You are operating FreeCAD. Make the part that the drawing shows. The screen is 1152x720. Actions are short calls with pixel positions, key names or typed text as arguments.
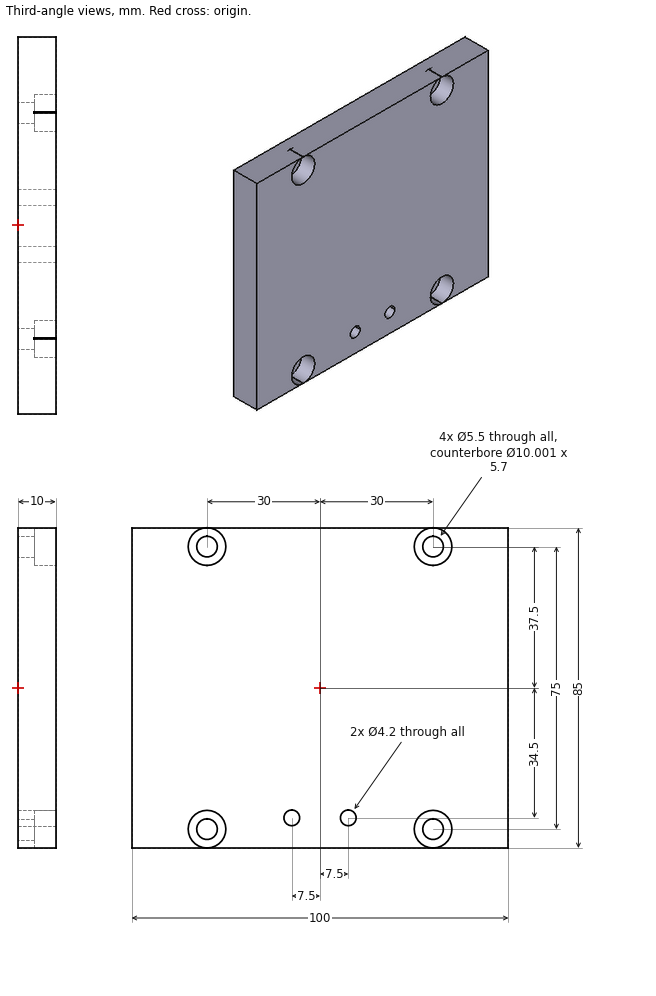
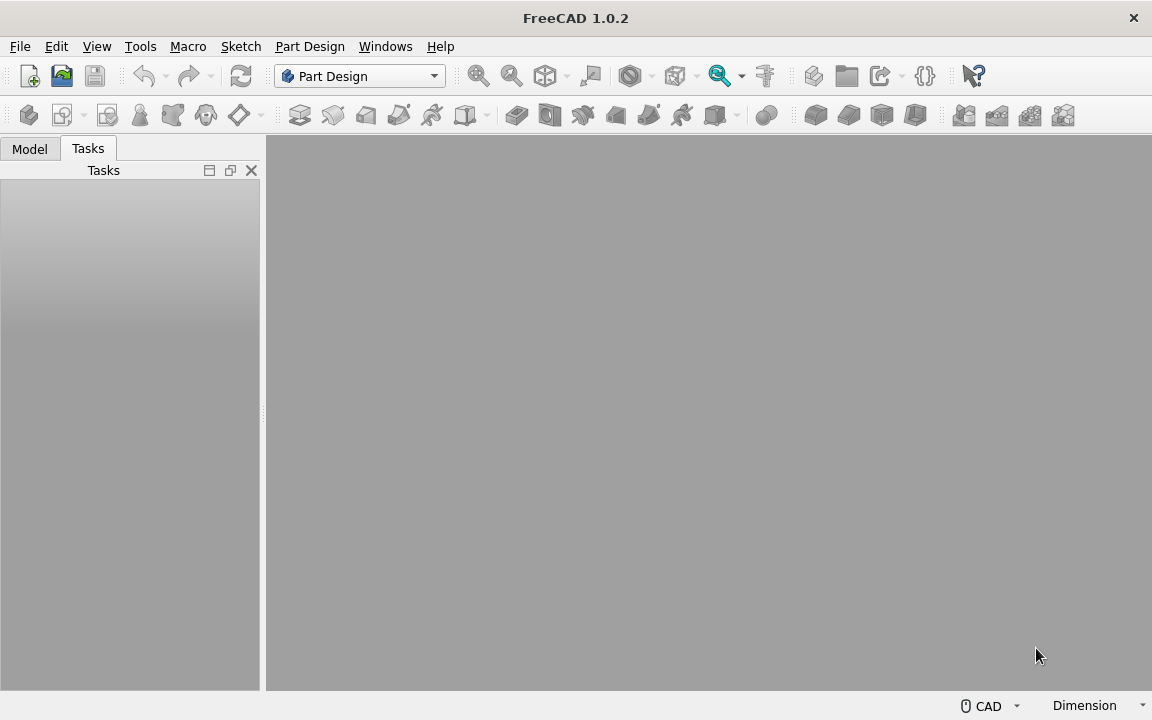
click(29, 76)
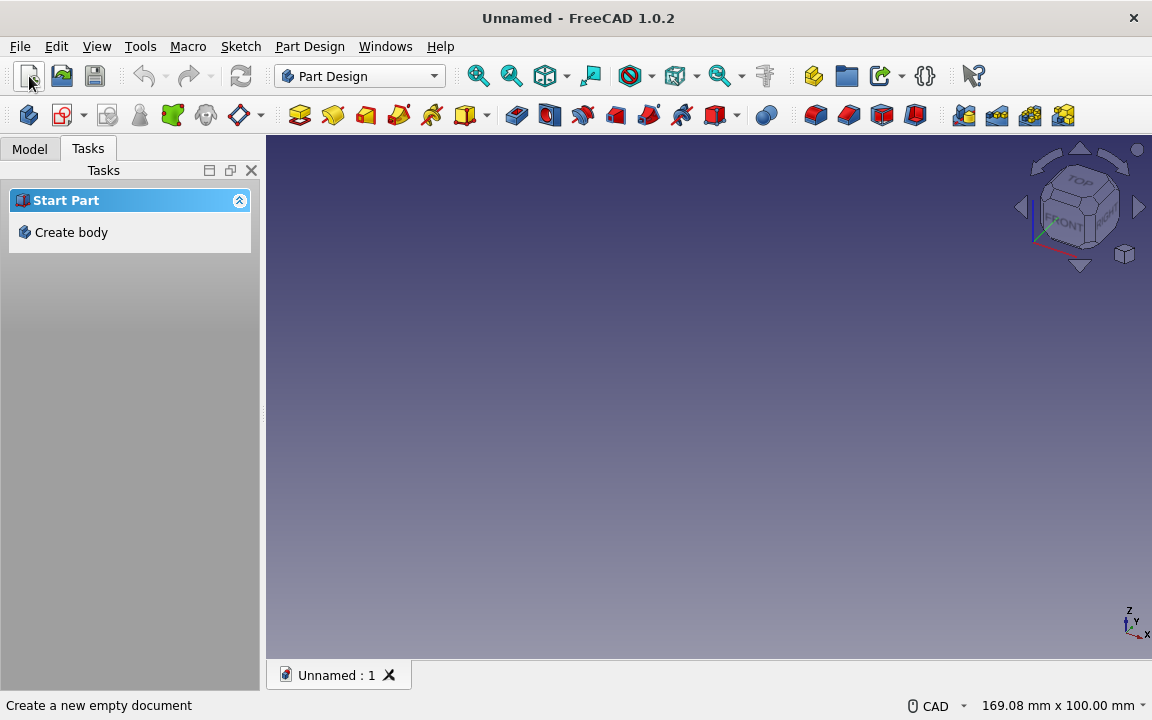
click(62, 116)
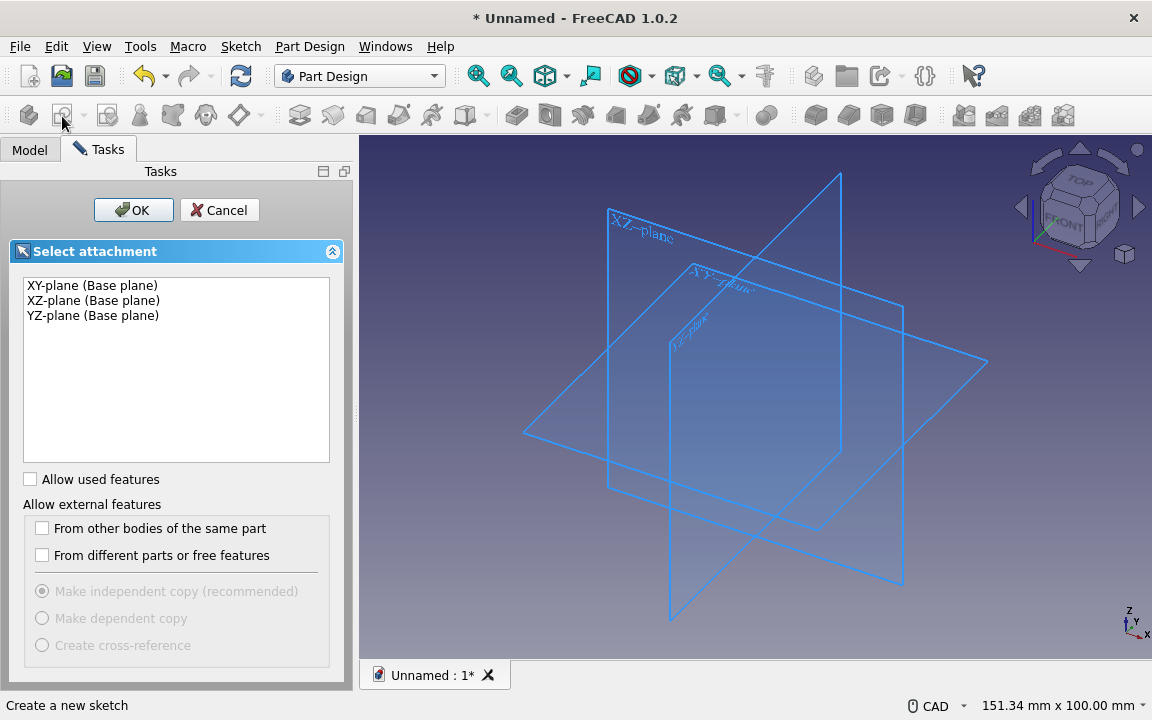
click(84, 316)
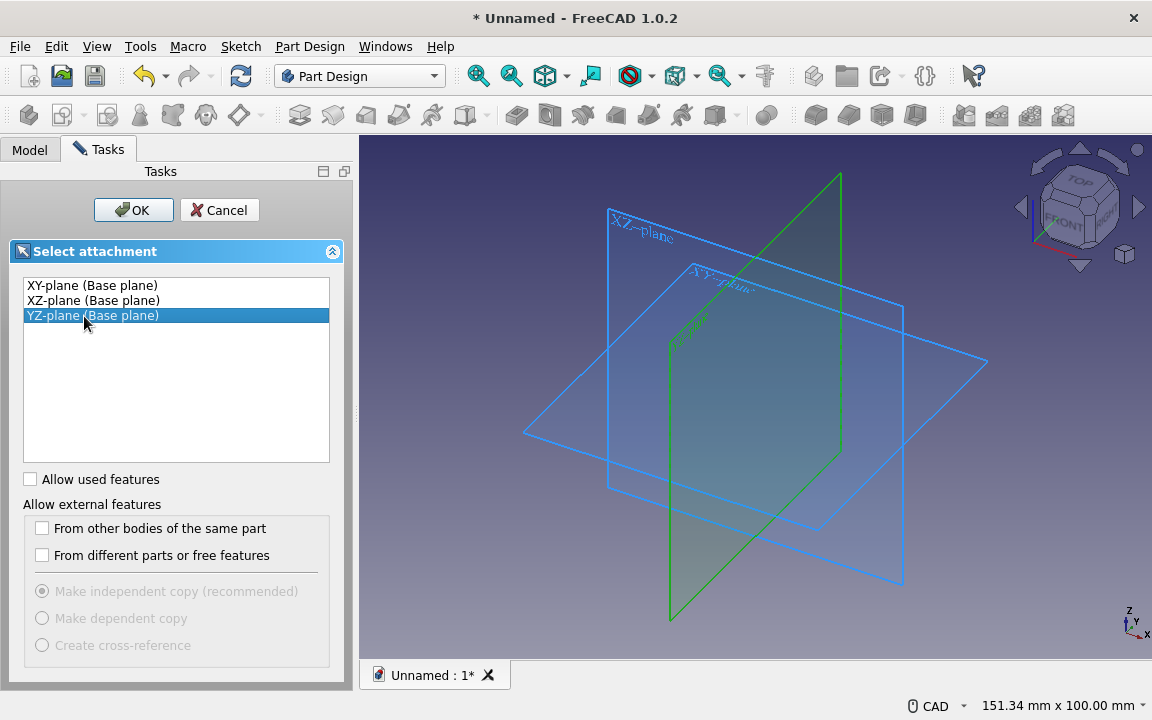
click(134, 210)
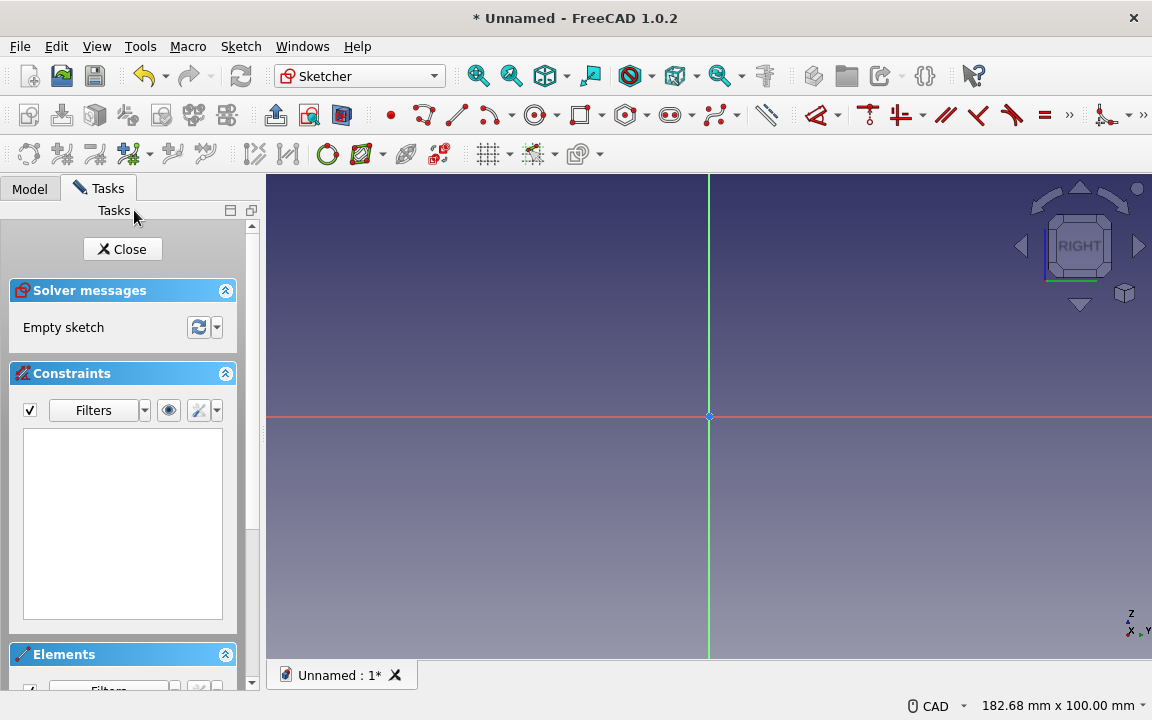
scroll(501, 416, down, 2)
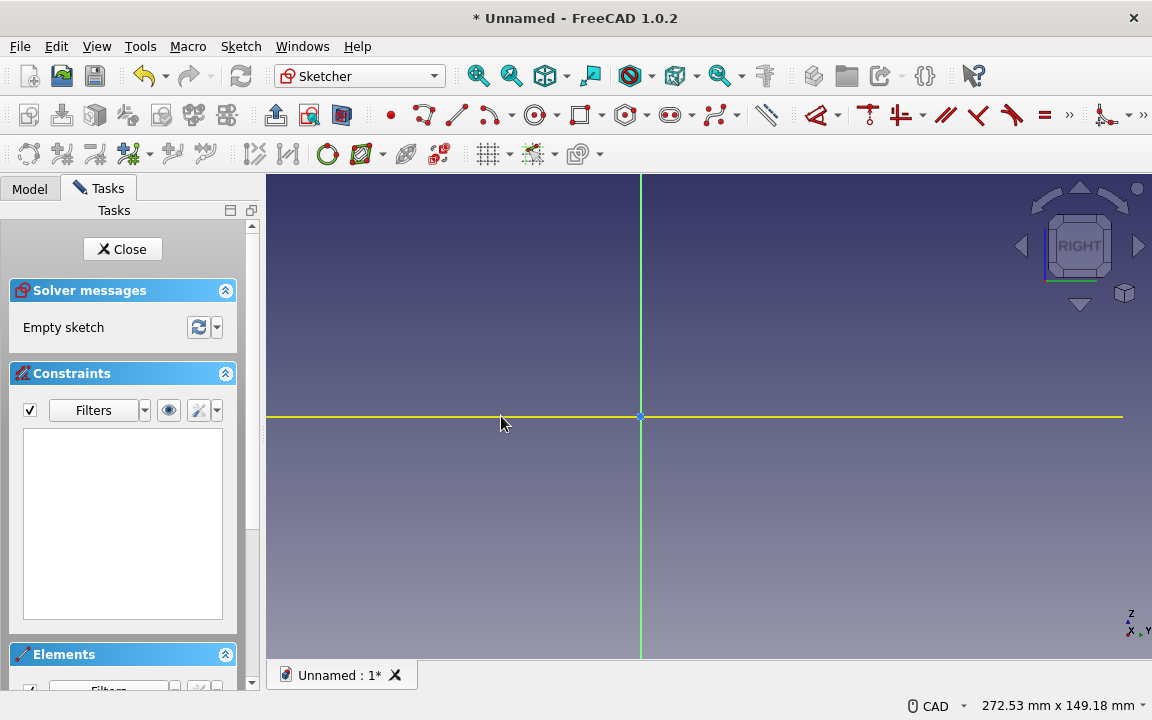
key(g)
key(v)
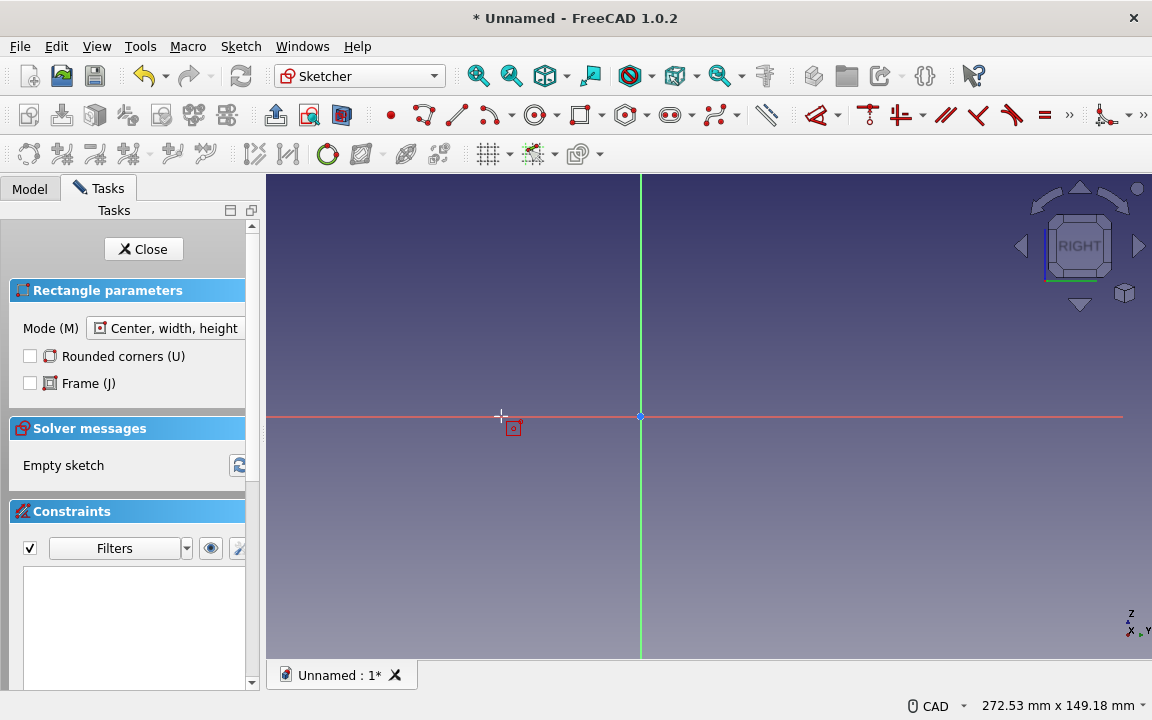
click(641, 416)
click(803, 278)
key(Escape)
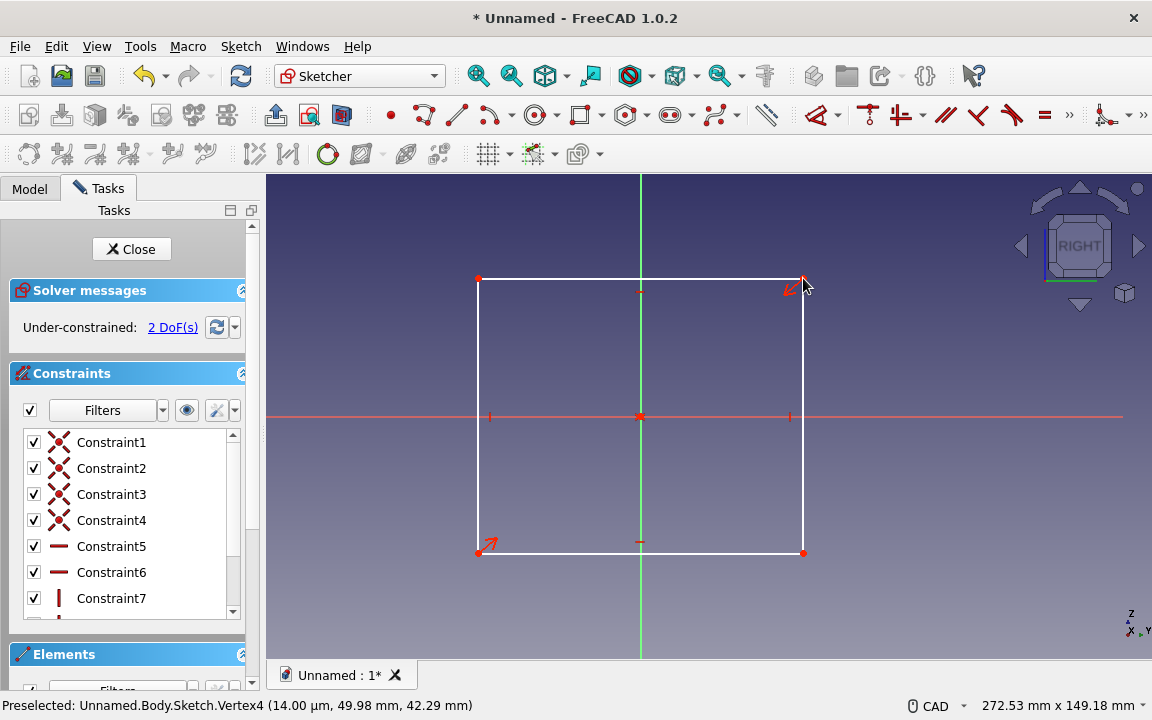
click(816, 116)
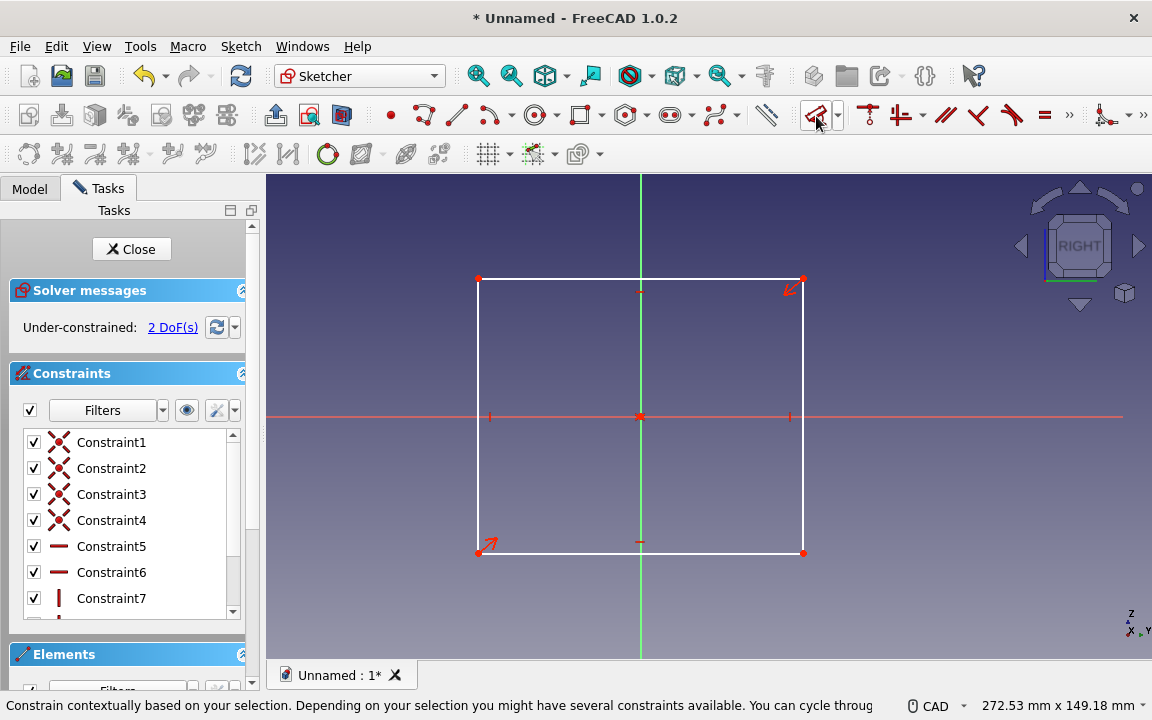
click(803, 471)
click(837, 353)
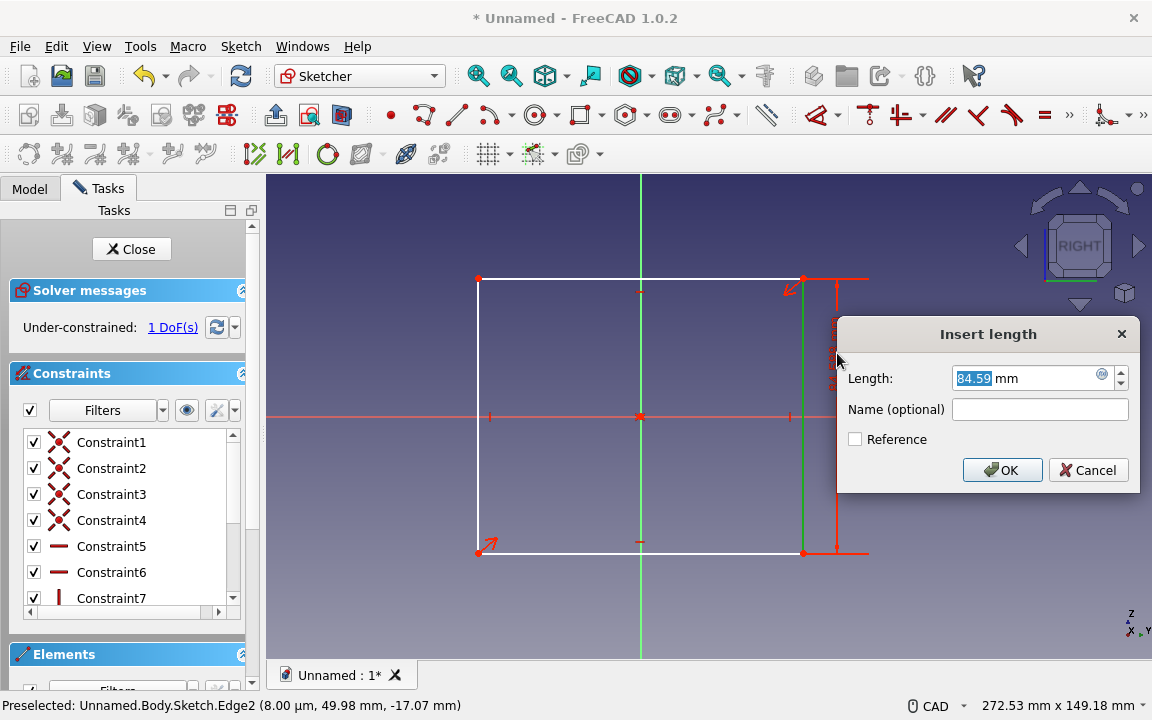
text(85)
key(Return)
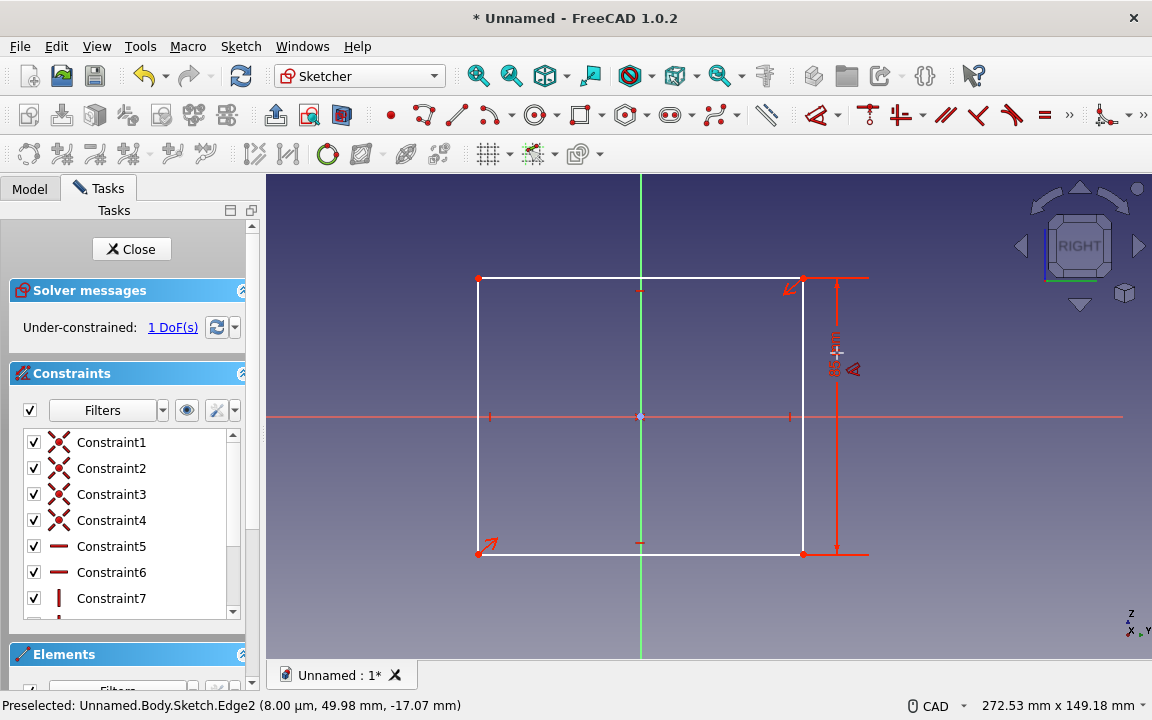
click(576, 555)
click(566, 589)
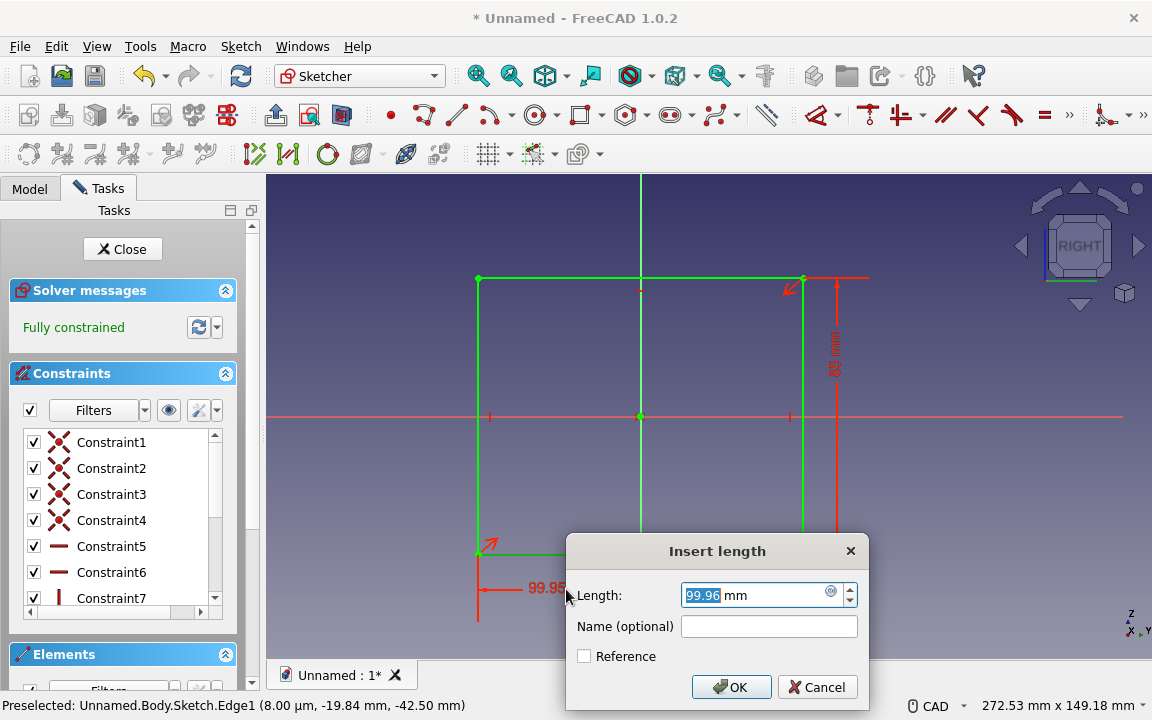
text(100)
key(Return)
key(Escape)